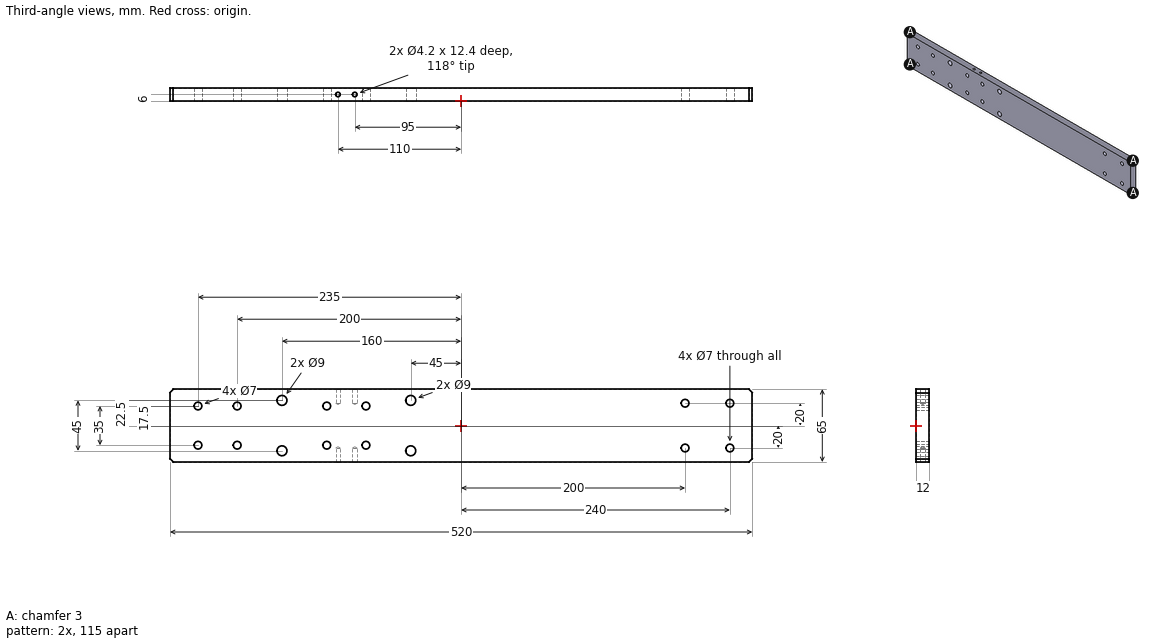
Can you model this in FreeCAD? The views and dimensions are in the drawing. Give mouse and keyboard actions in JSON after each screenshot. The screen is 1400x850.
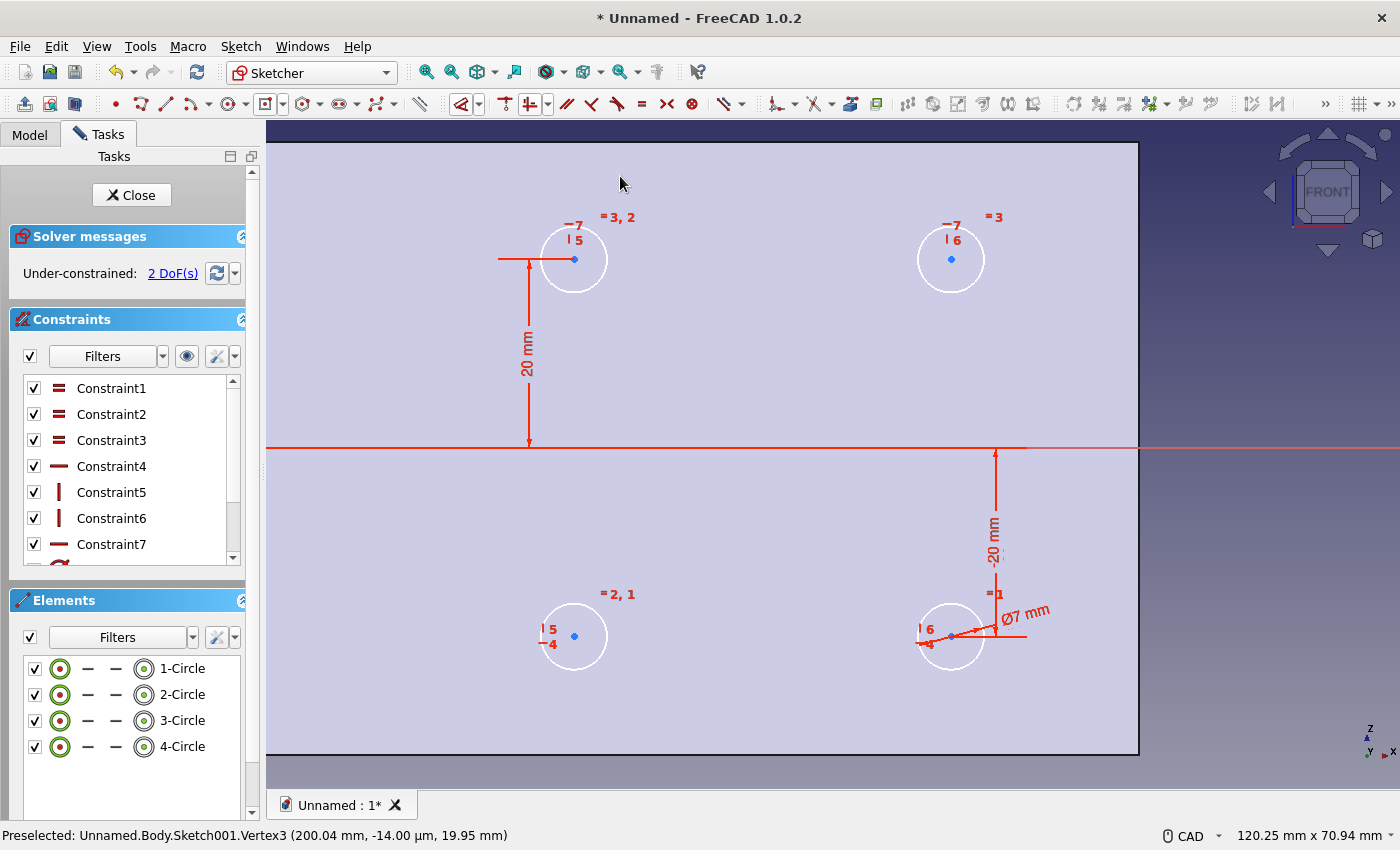
{"action": "left_click", "coordinate": [951, 637]}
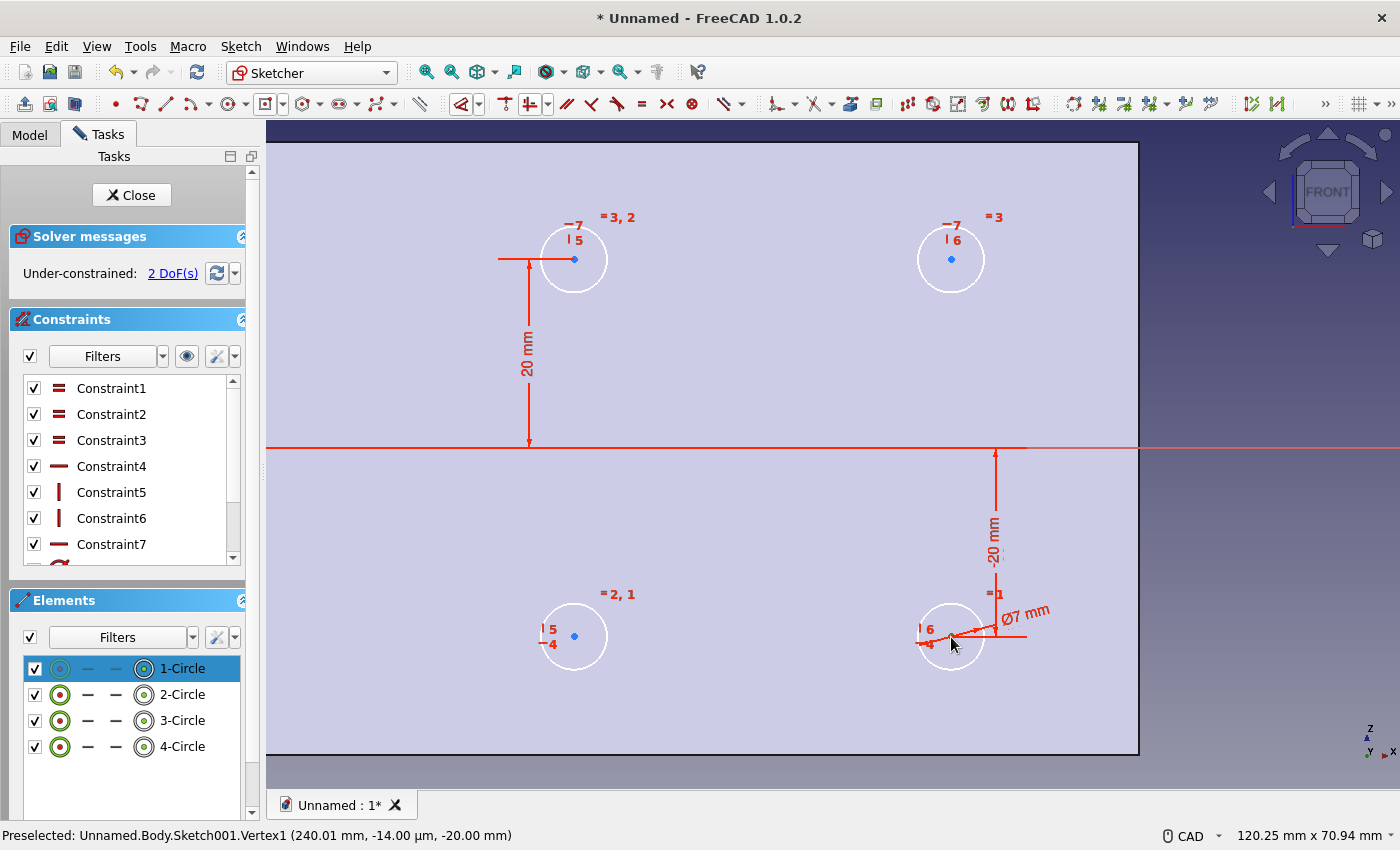
{"action": "left_click", "coordinate": [478, 104]}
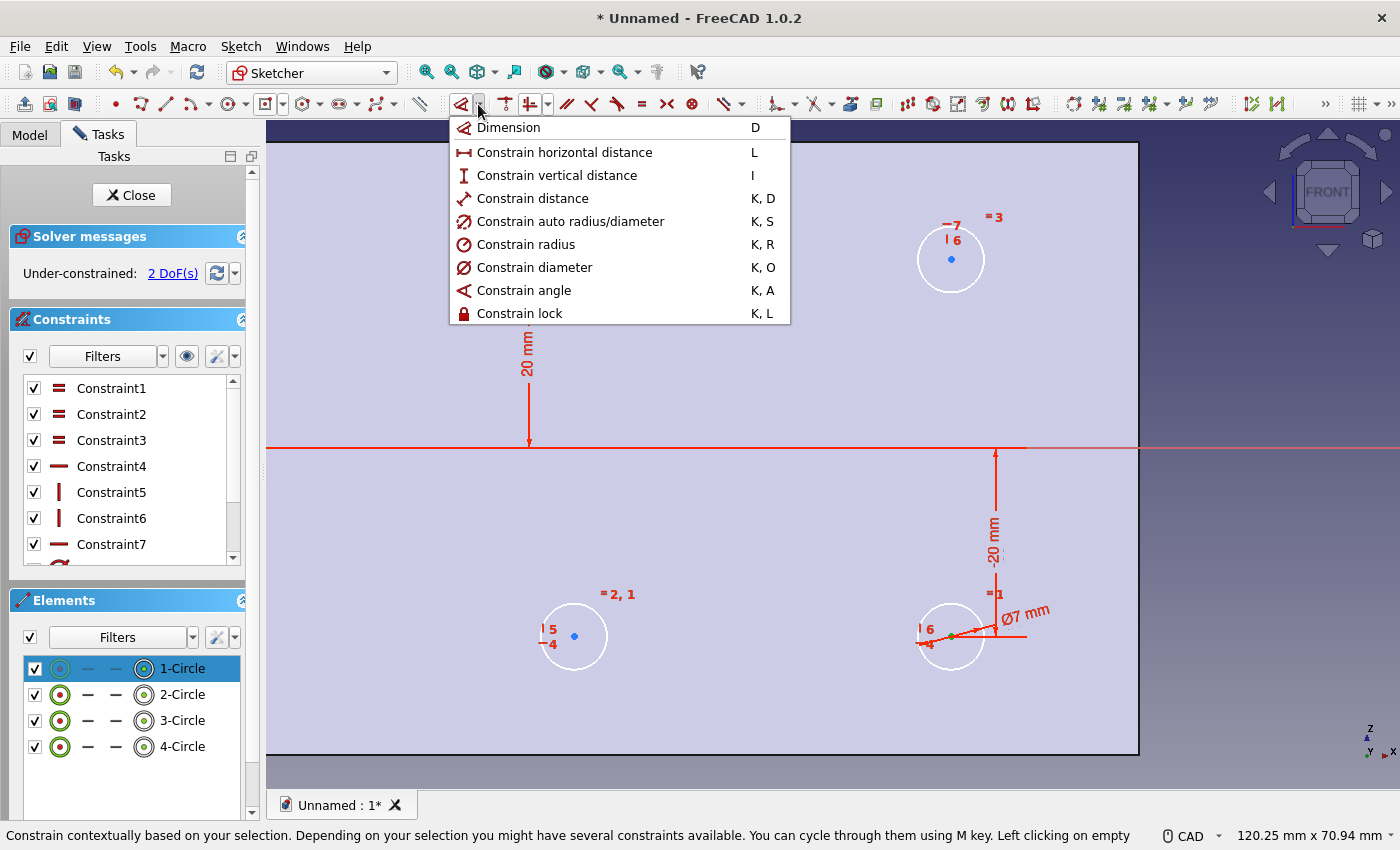
{"action": "left_click", "coordinate": [620, 152]}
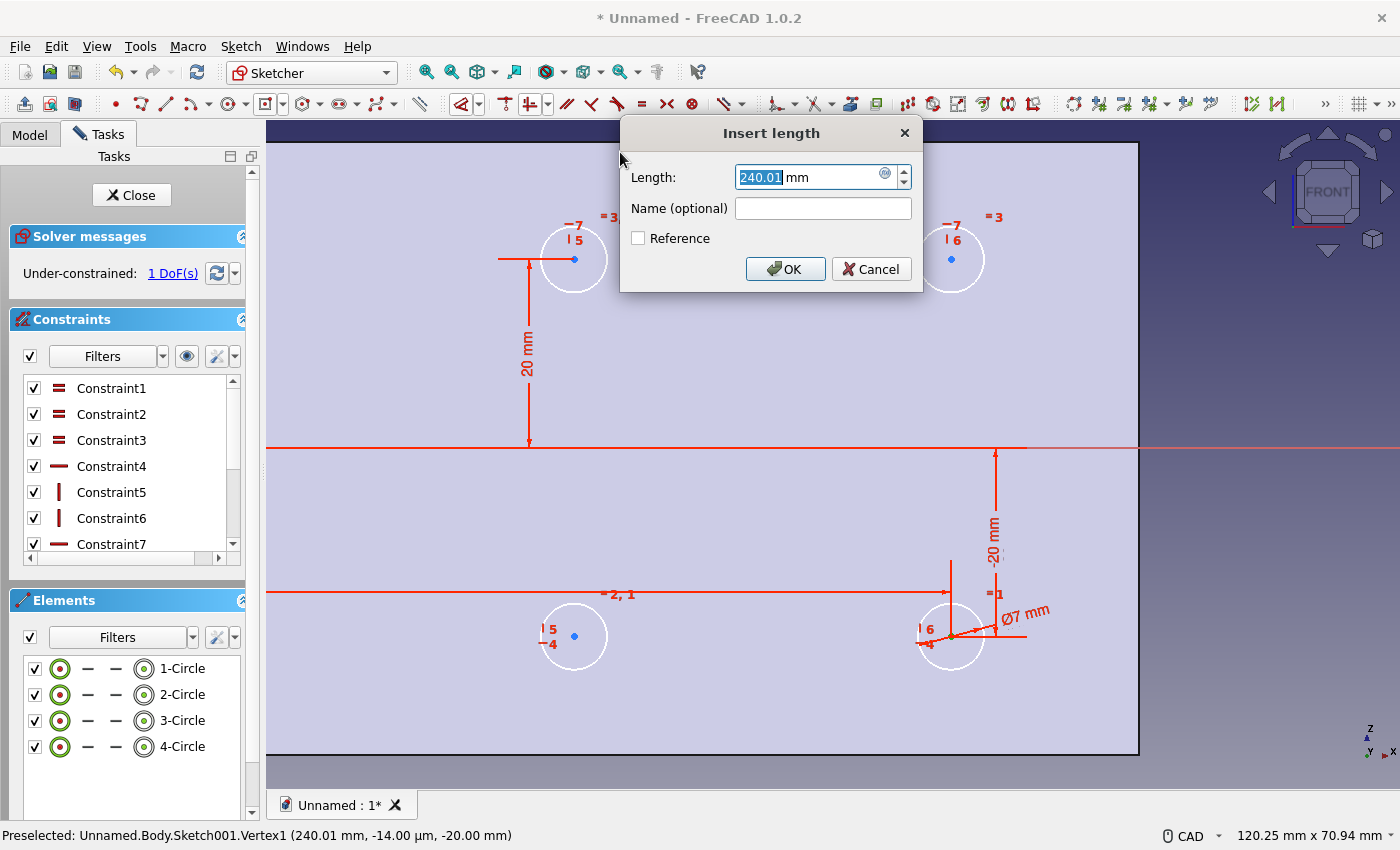
{"action": "type", "text": "240"}
{"action": "key", "text": "Return"}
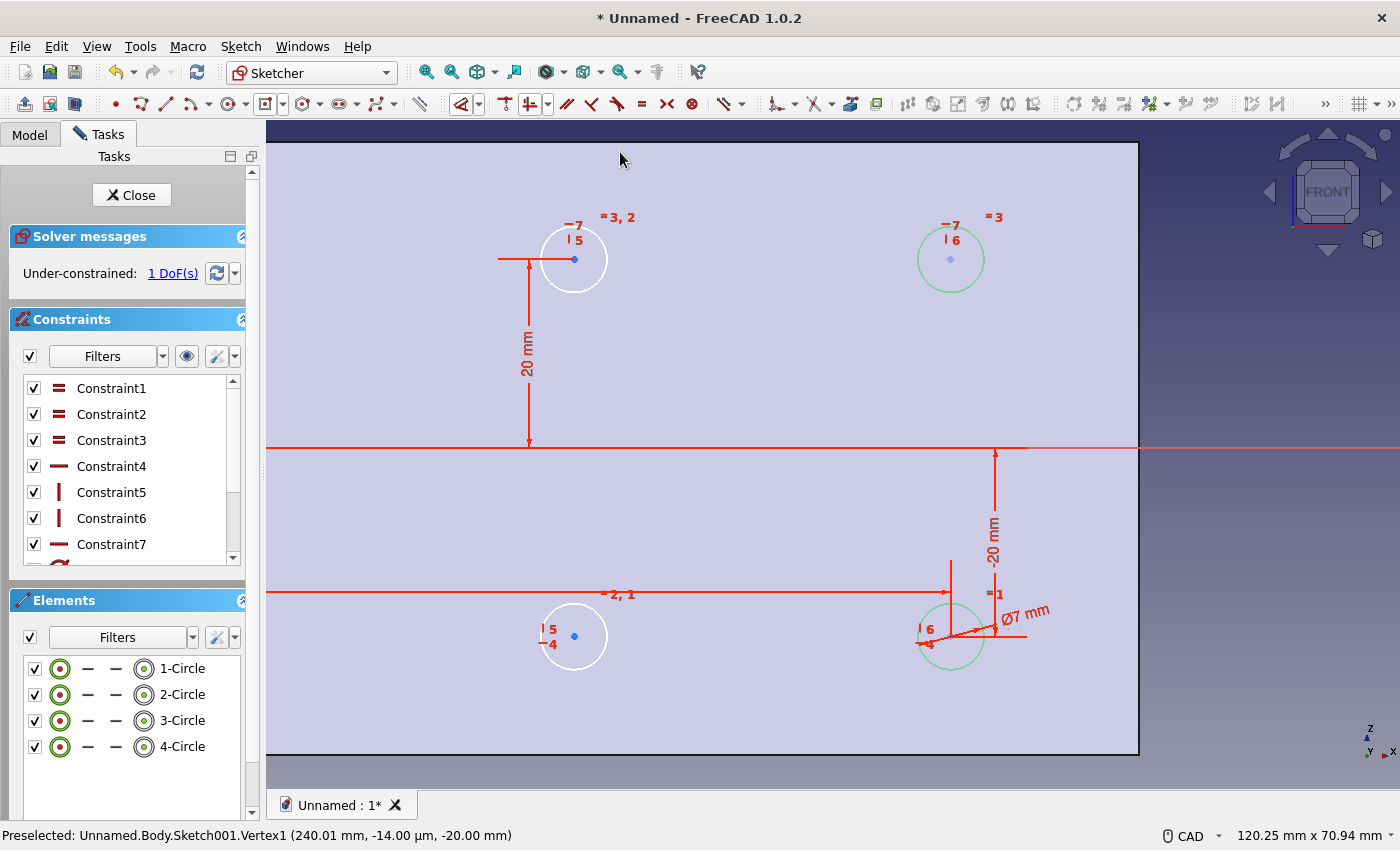
{"action": "left_click", "coordinate": [574, 637]}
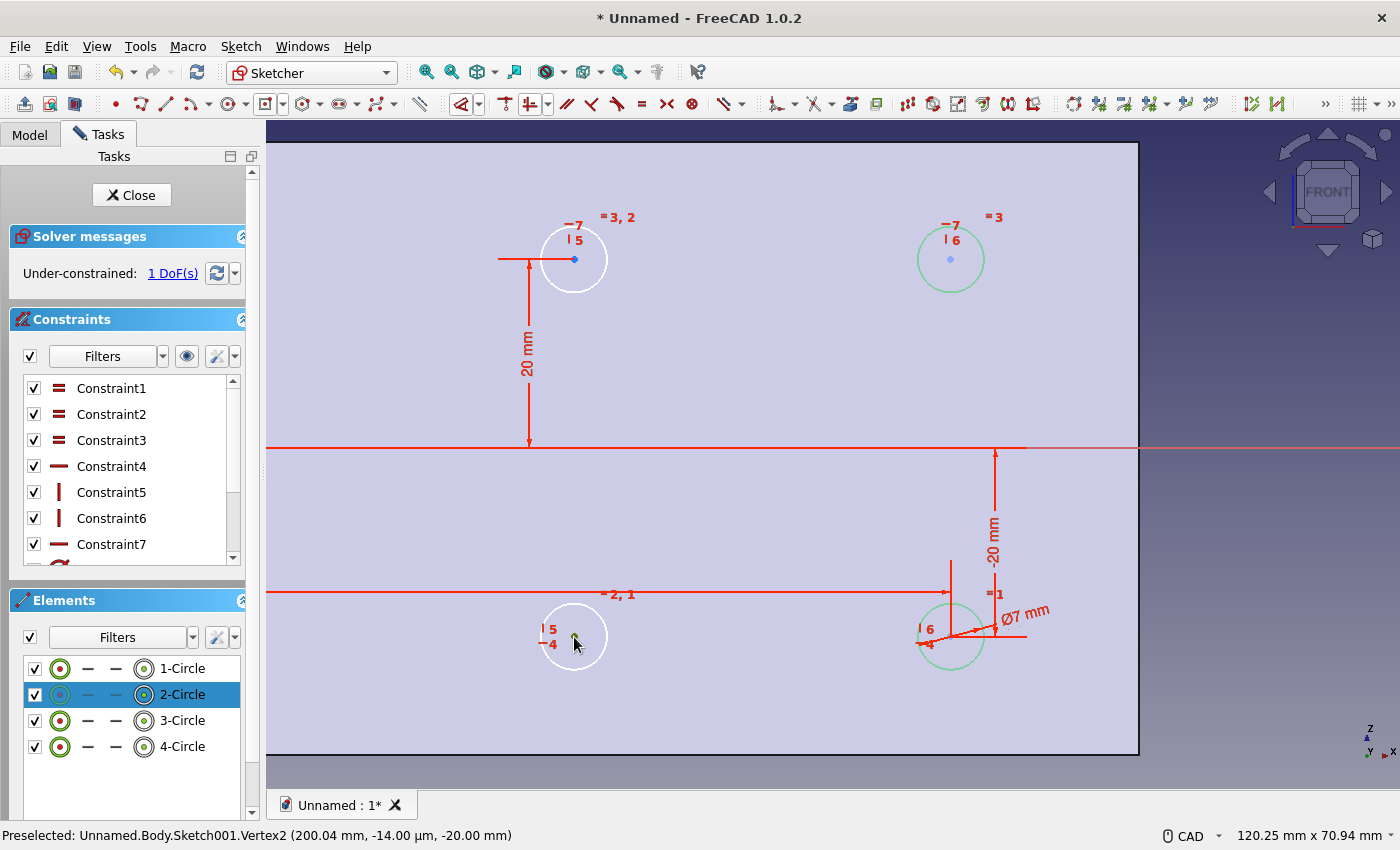
{"action": "key", "text": "l"}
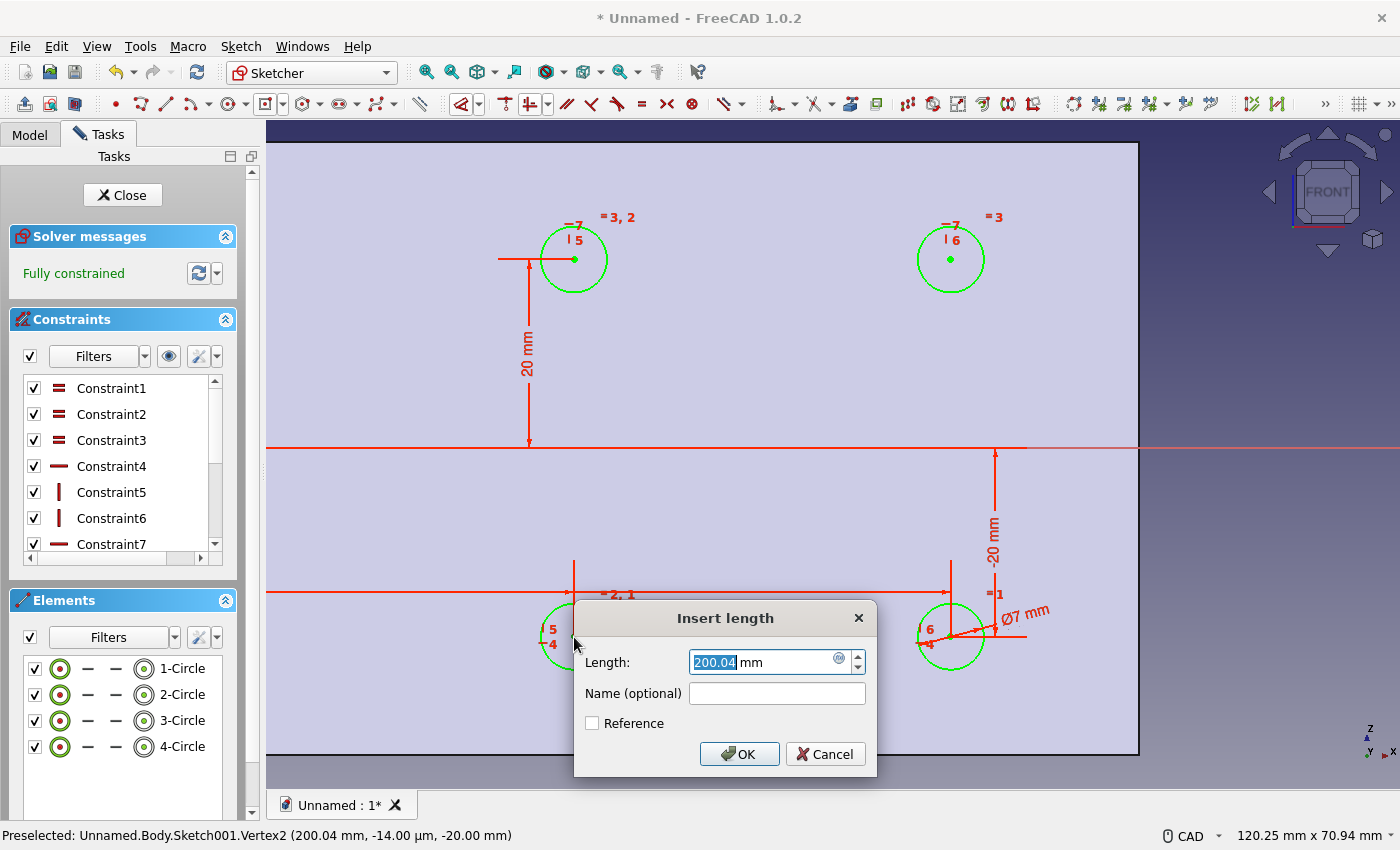
{"action": "type", "text": "200"}
{"action": "key", "text": "Return"}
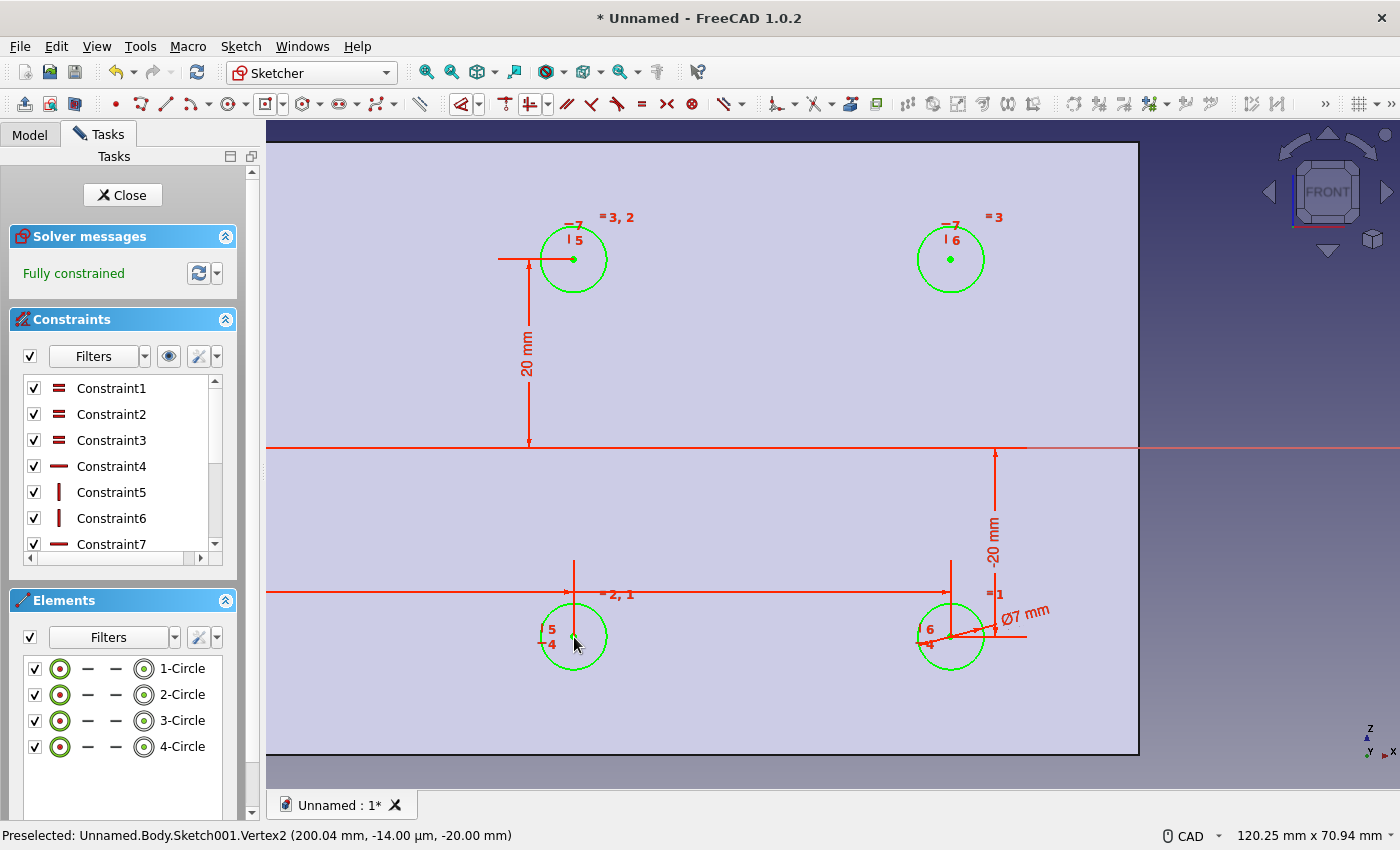
{"action": "left_click", "coordinate": [123, 195]}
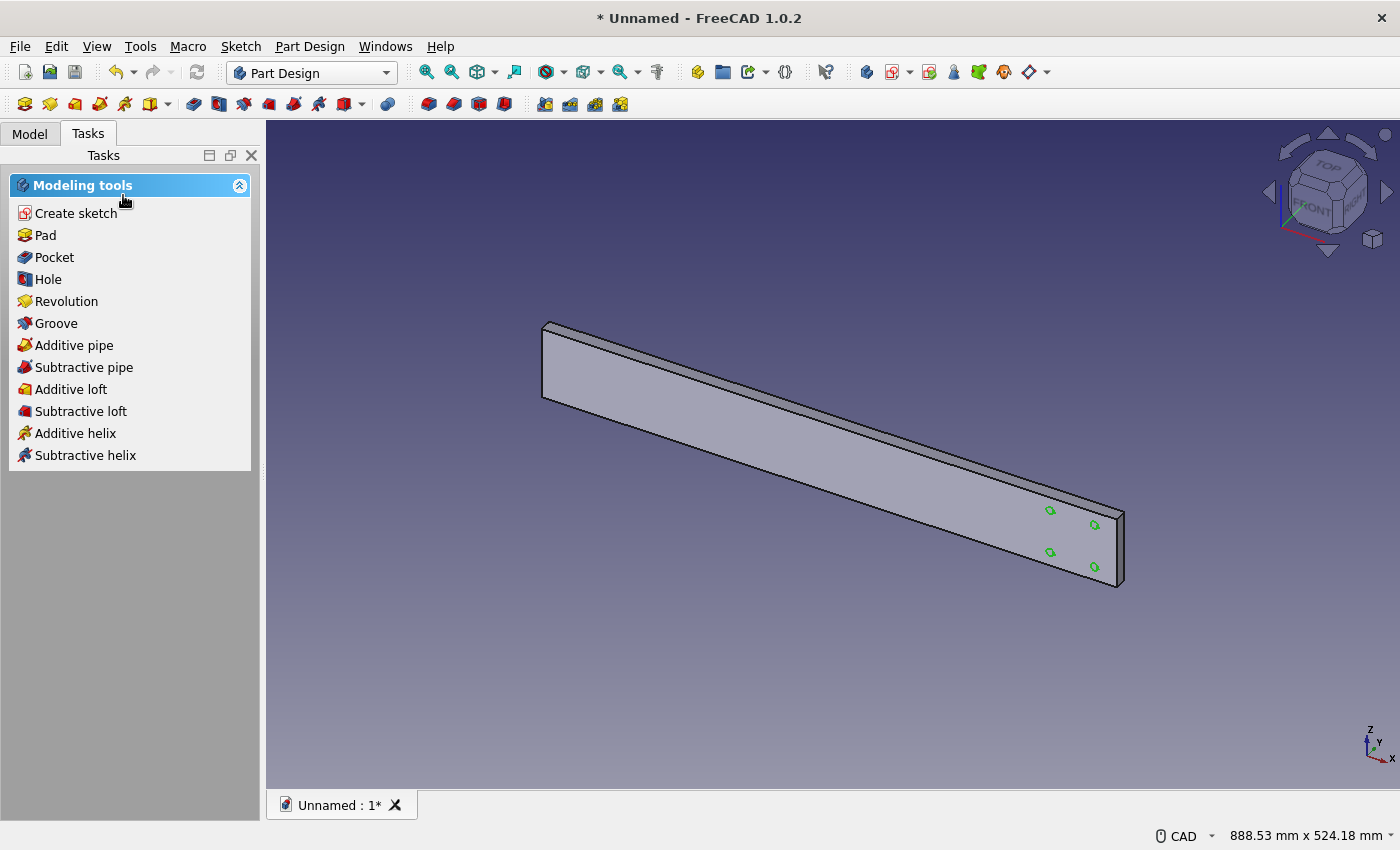
{"action": "left_click", "coordinate": [219, 104]}